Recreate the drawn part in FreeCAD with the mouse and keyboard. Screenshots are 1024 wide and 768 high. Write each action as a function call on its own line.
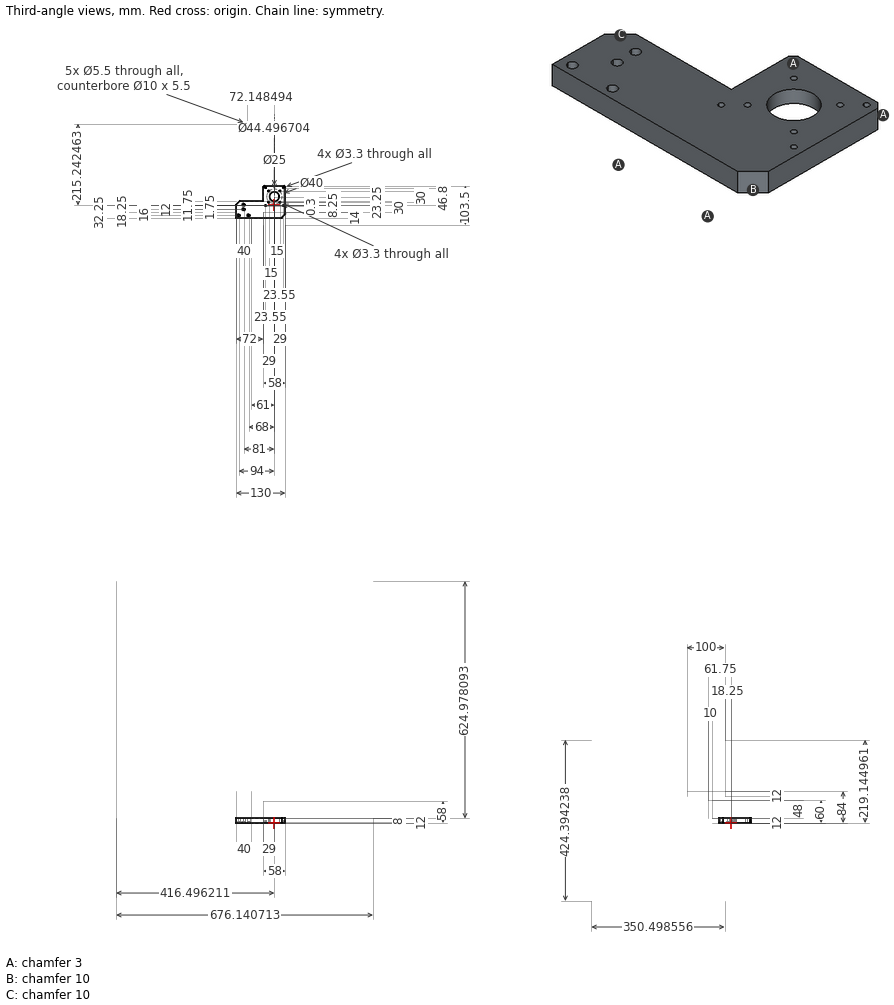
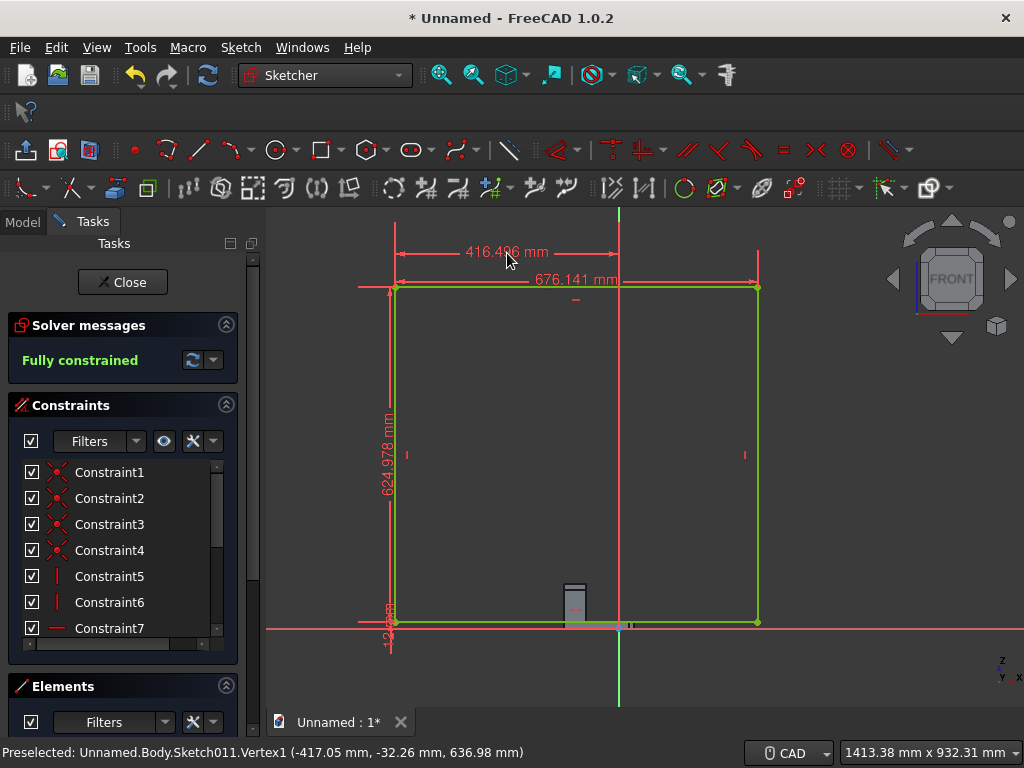
click(123, 282)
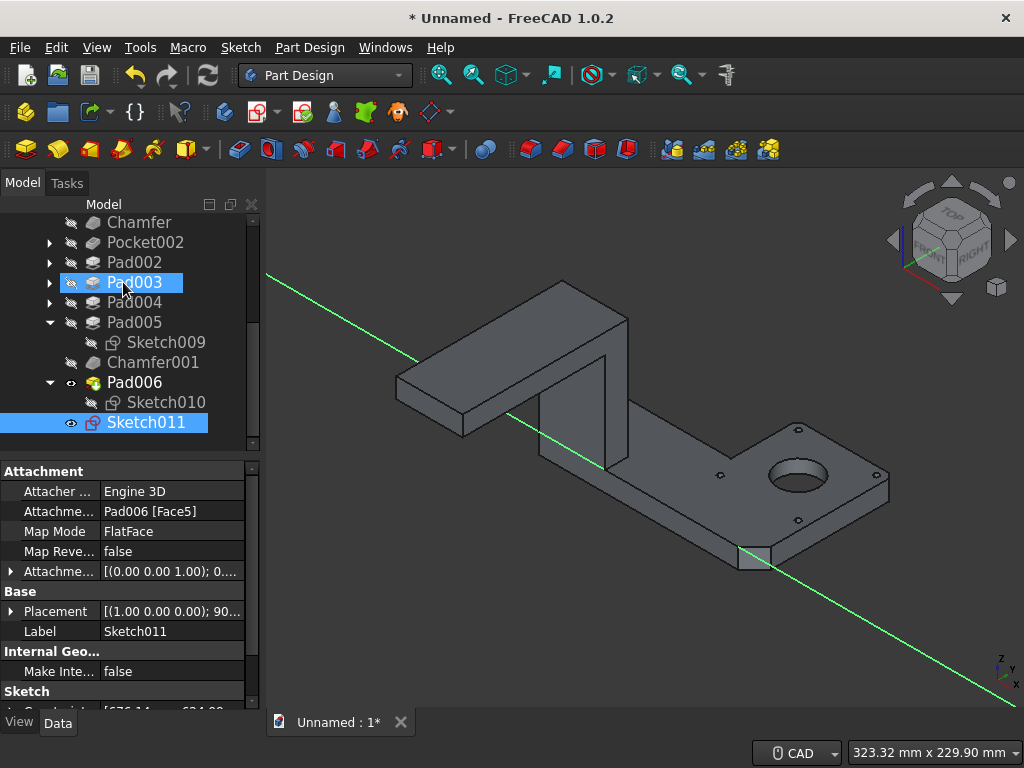
click(240, 150)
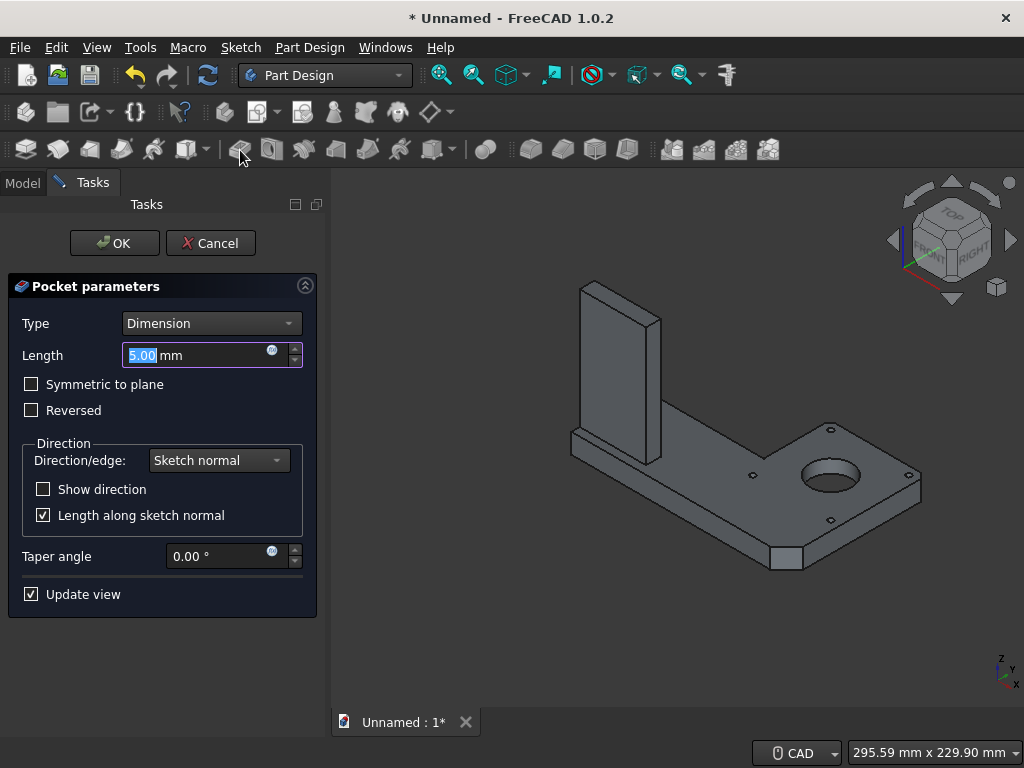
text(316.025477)
key(Tab)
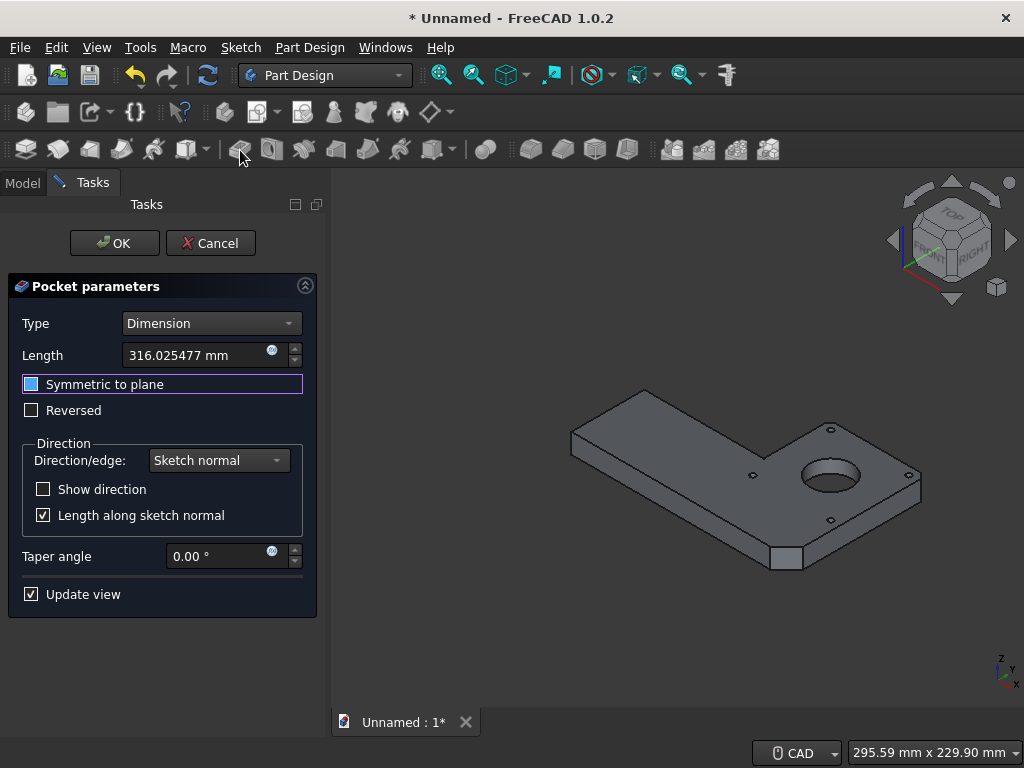
click(30, 384)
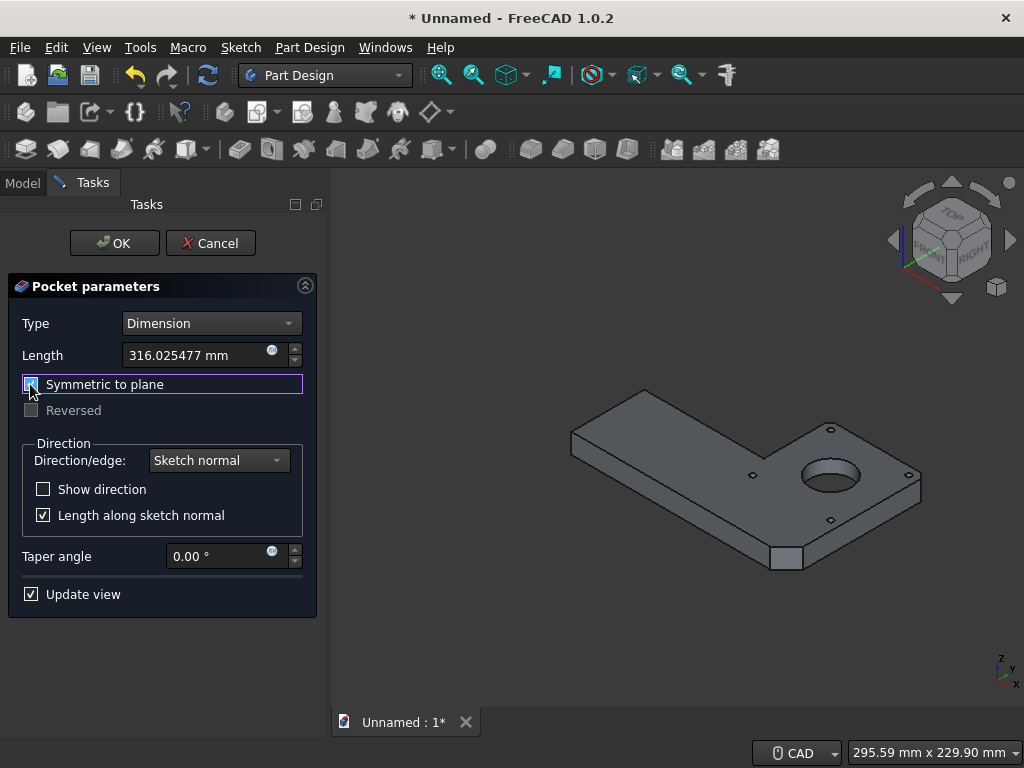
click(115, 243)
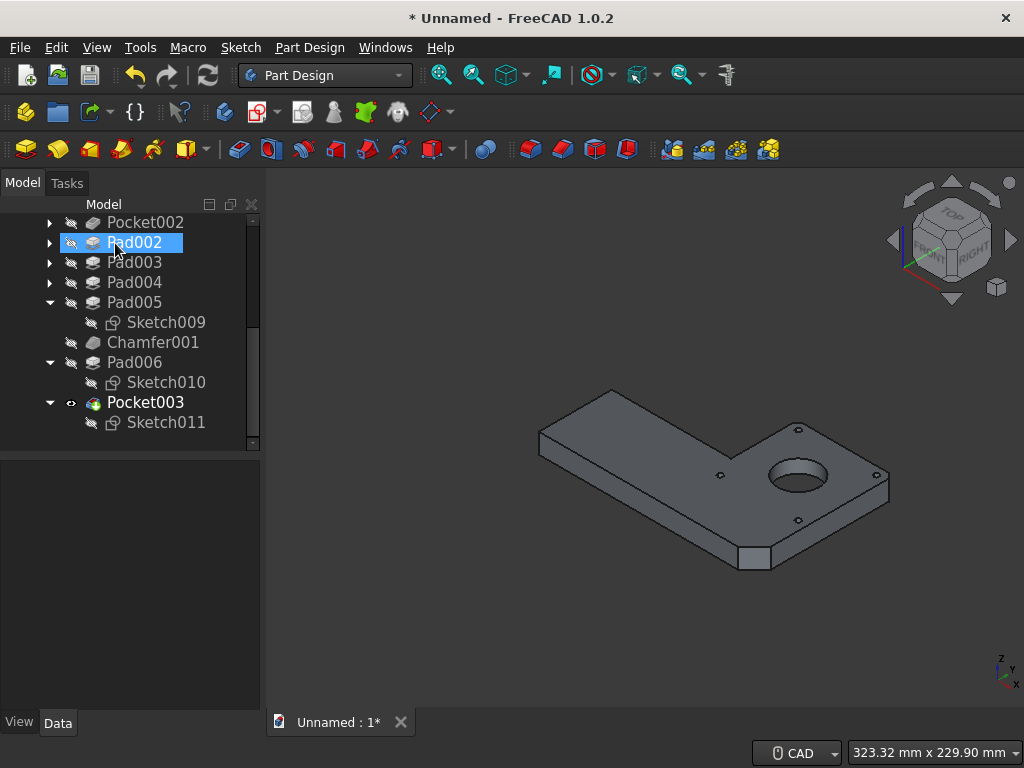
key(5)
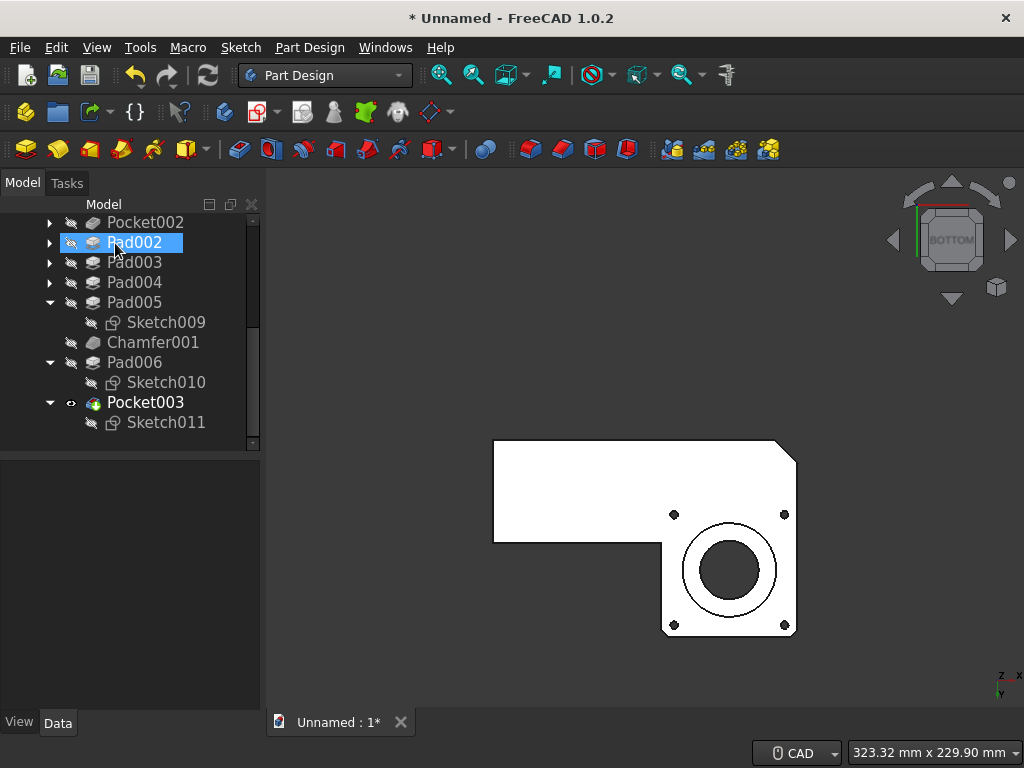
click(442, 76)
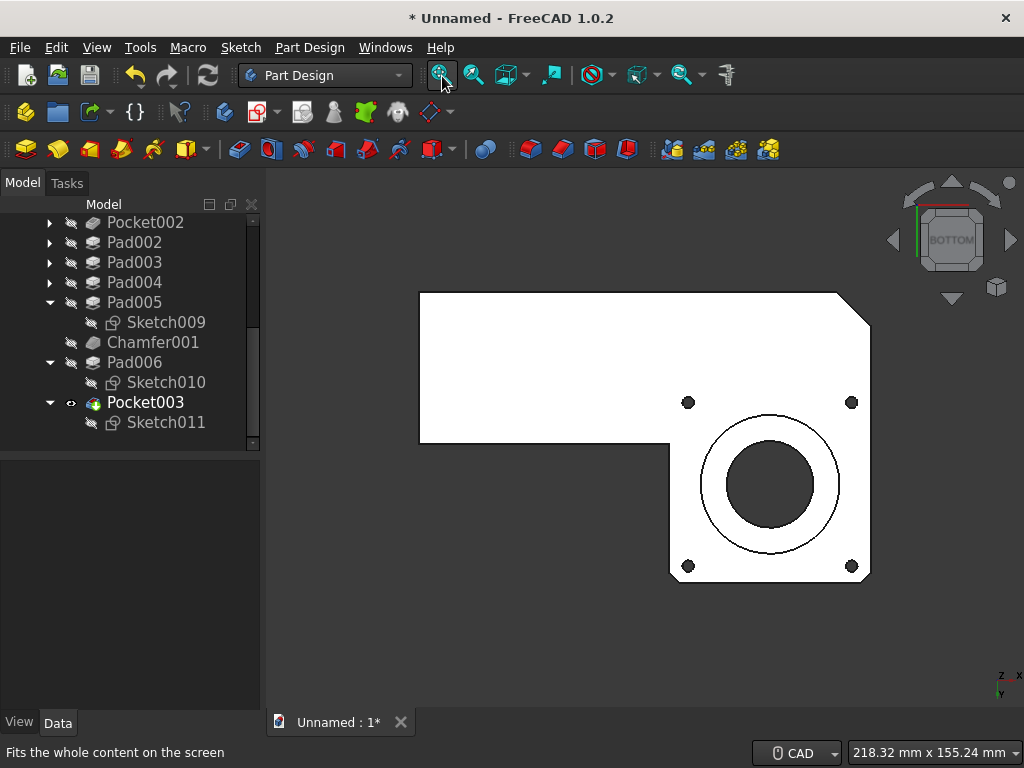
click(581, 353)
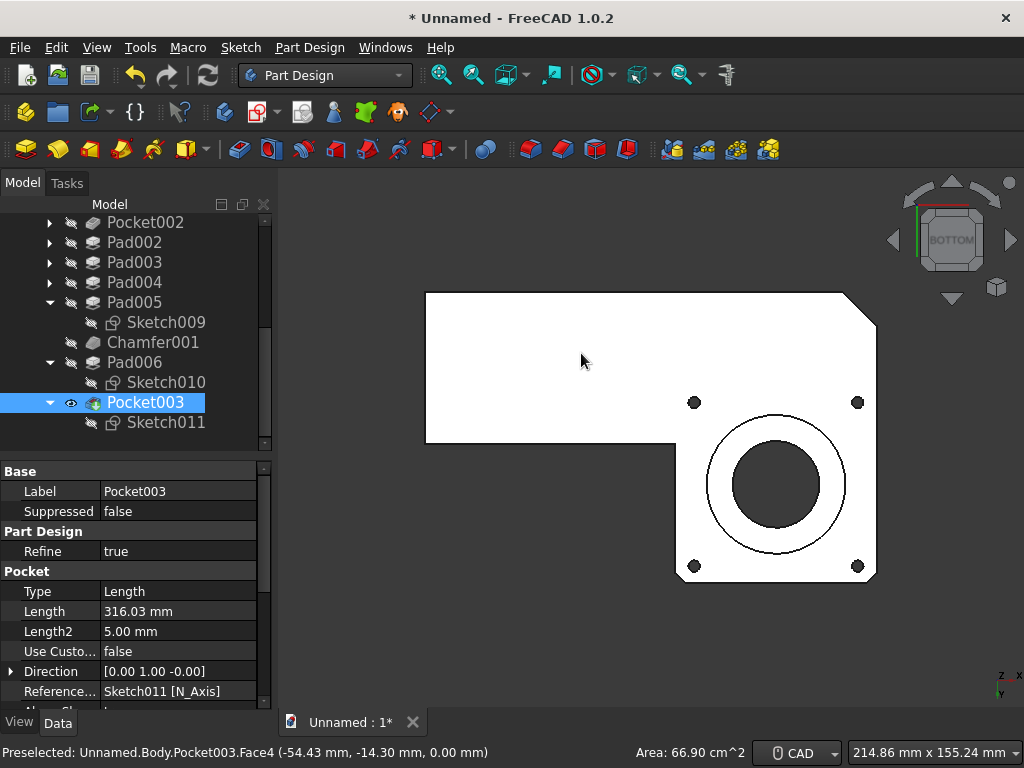
click(258, 112)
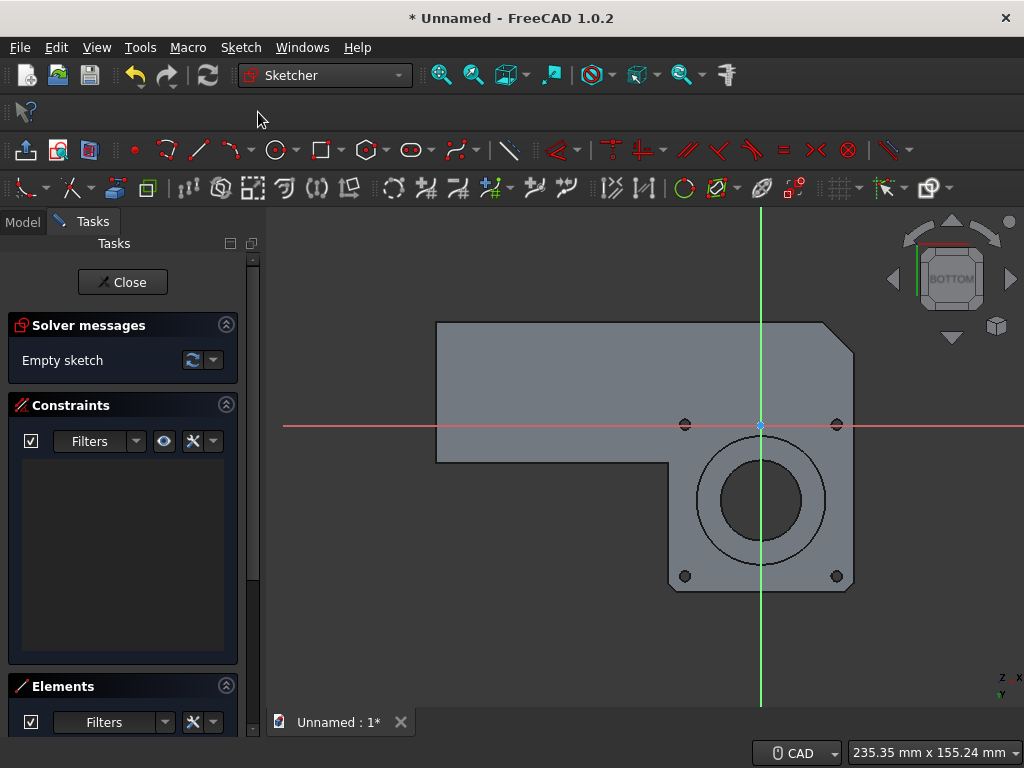
scroll(560, 298, down, 5)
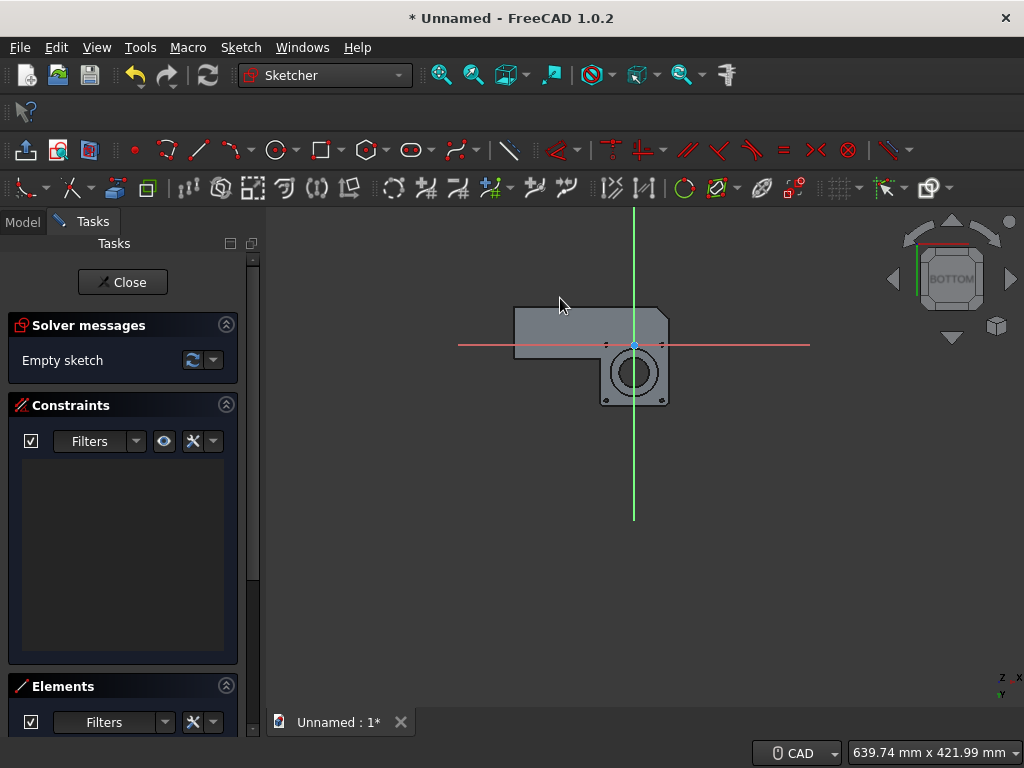
click(276, 150)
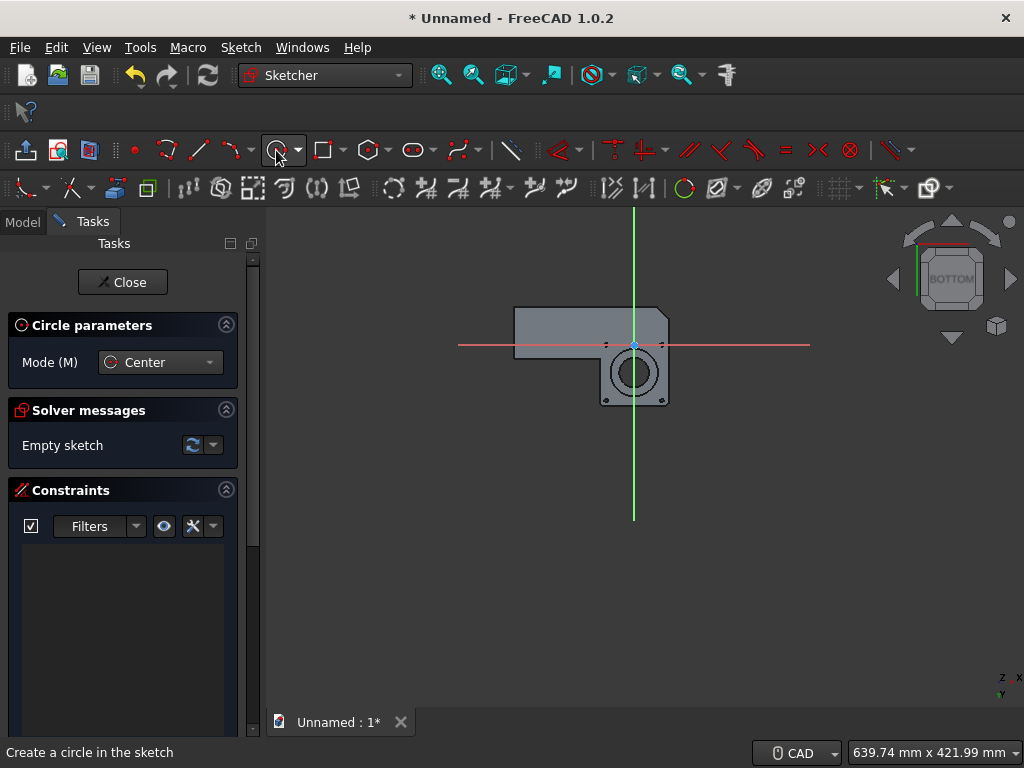
scroll(549, 600, up, 10)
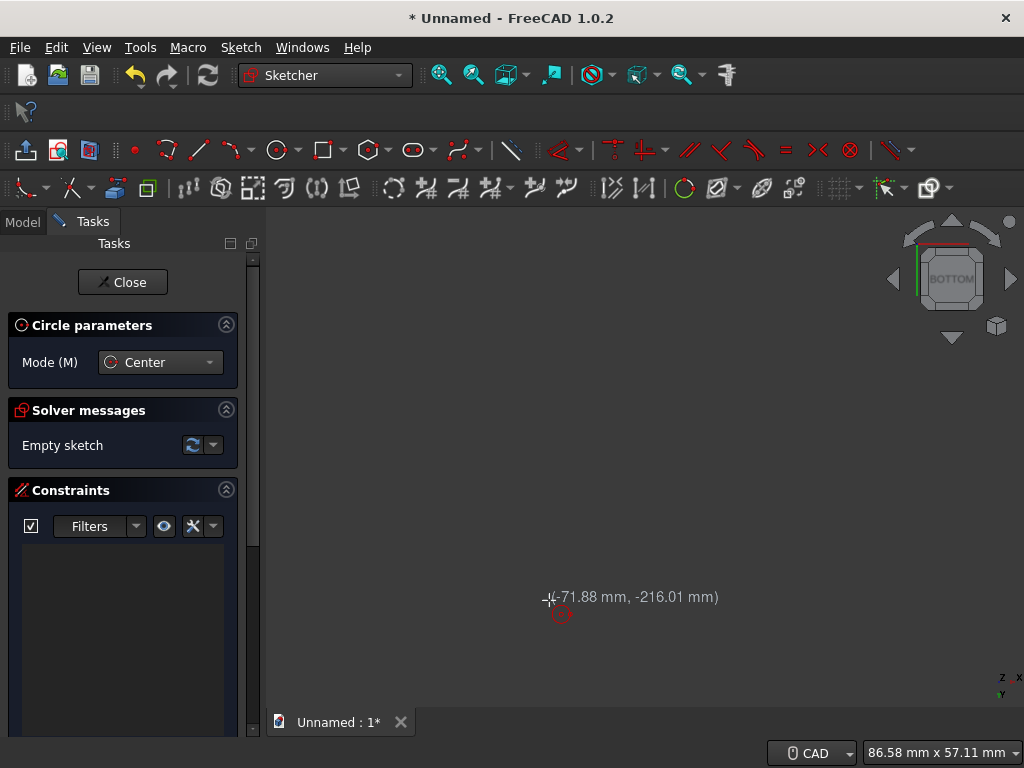
scroll(549, 601, down, 10)